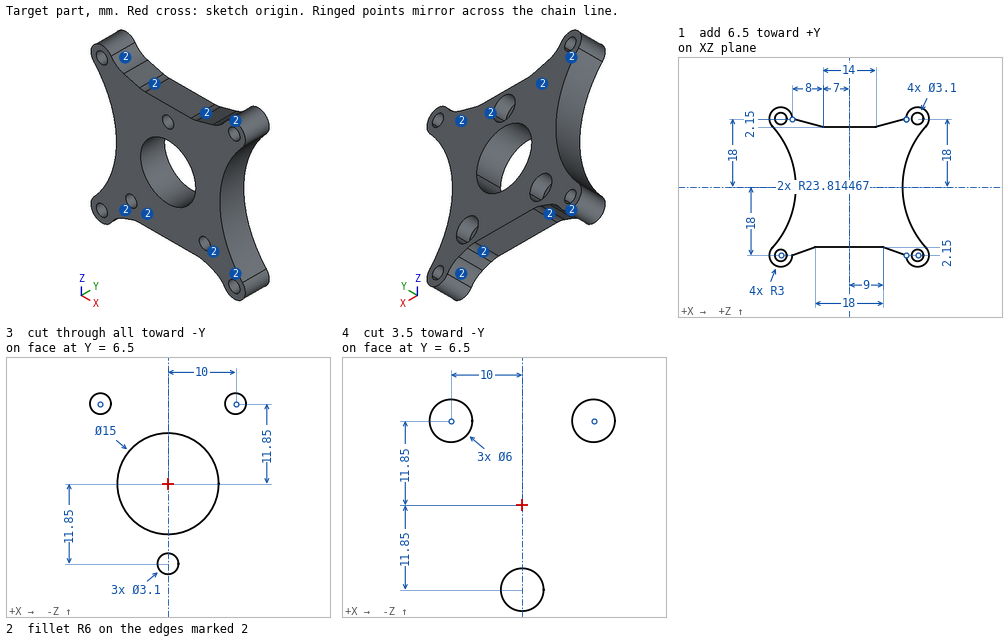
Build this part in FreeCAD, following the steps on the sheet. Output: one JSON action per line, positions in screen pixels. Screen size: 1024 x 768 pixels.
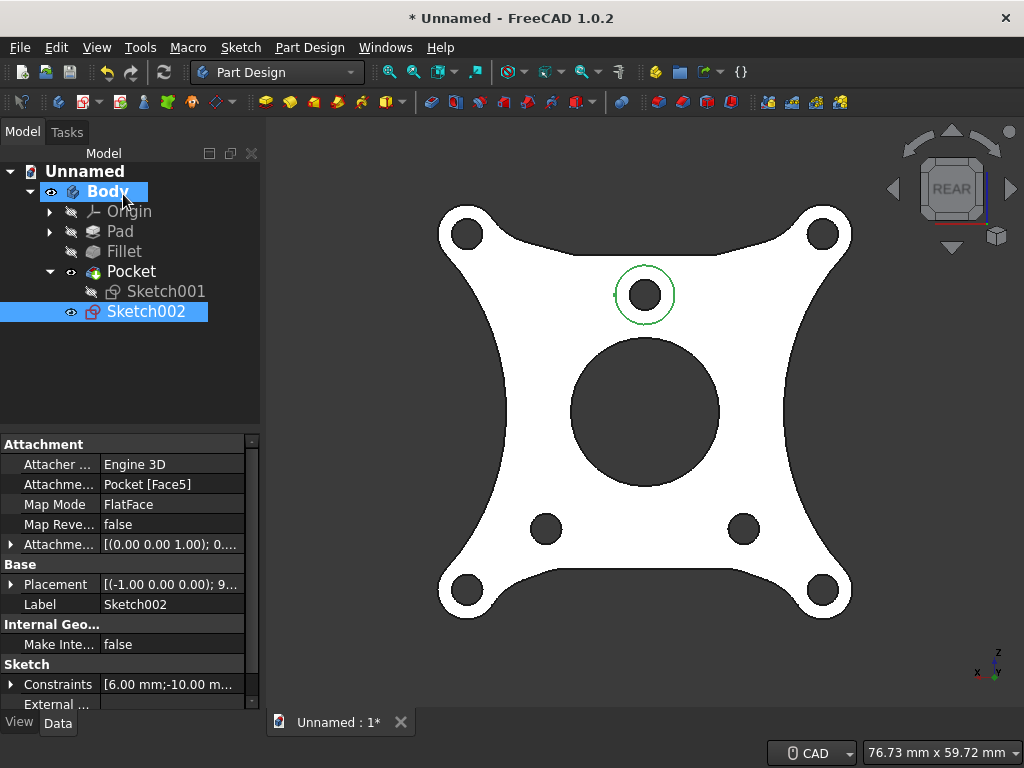
{"action": "left_click", "coordinate": [432, 102]}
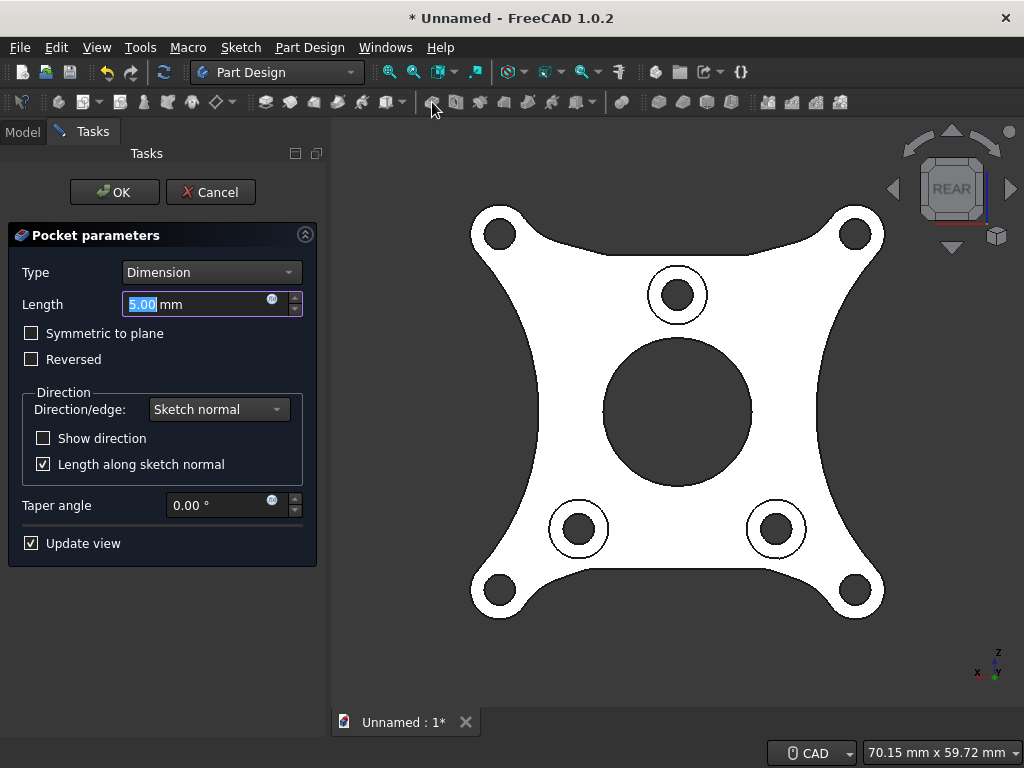
{"action": "type", "text": "3.5"}
{"action": "key", "text": "Tab"}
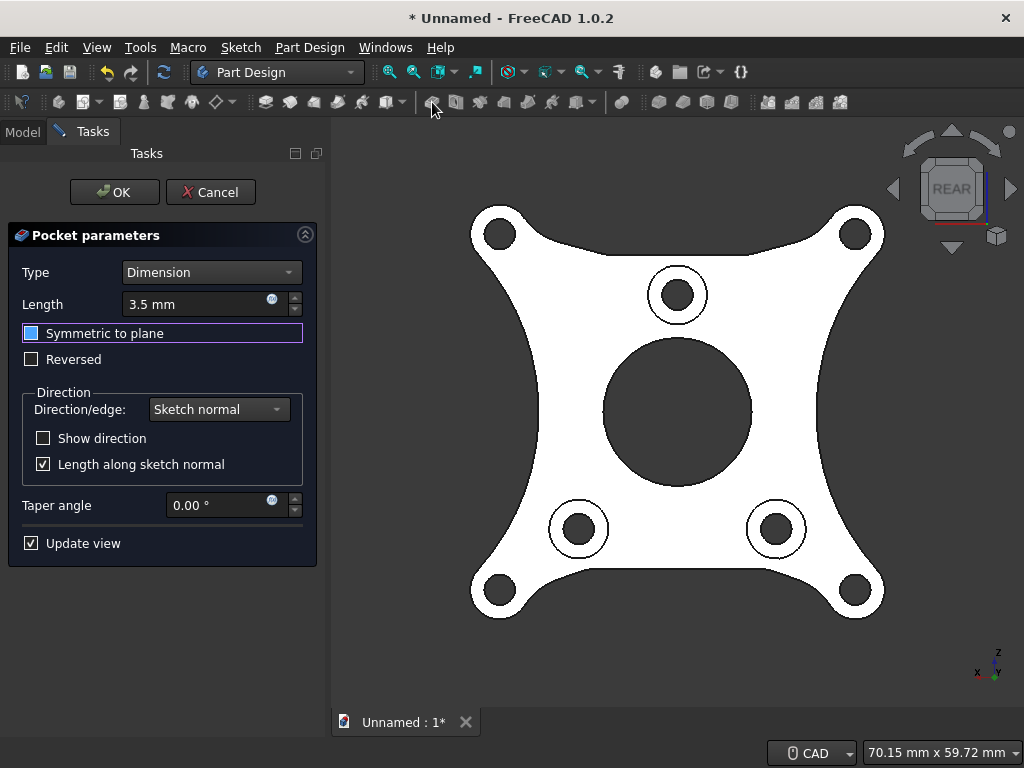
{"action": "left_click", "coordinate": [115, 192]}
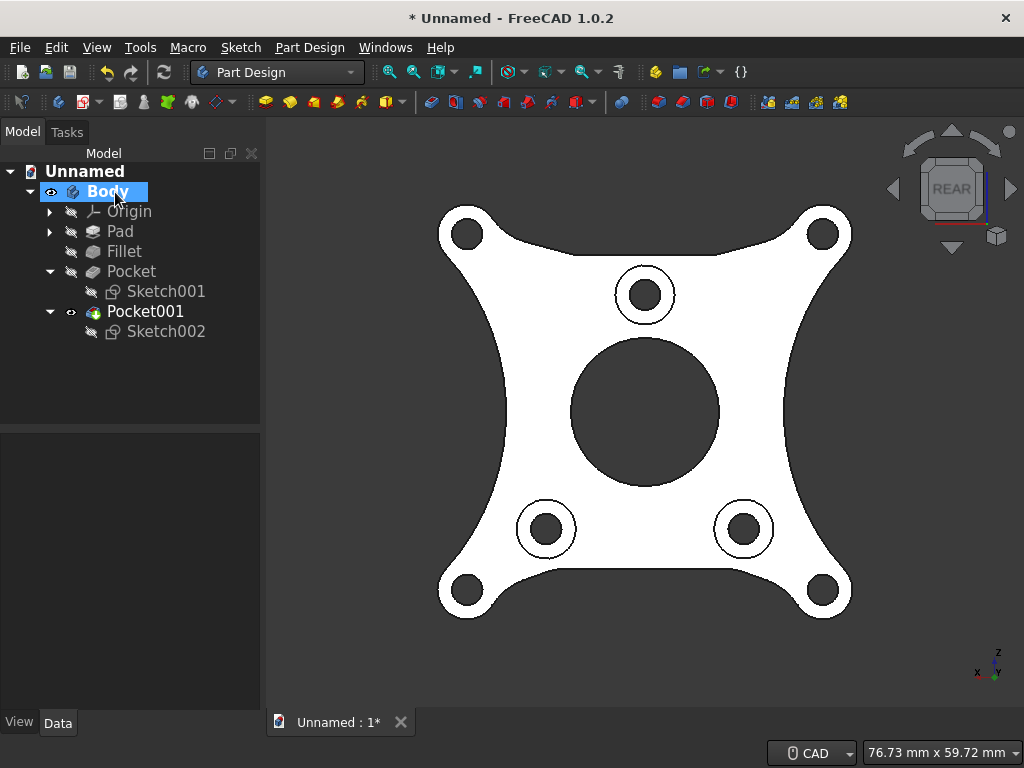
{"action": "key", "text": "0"}